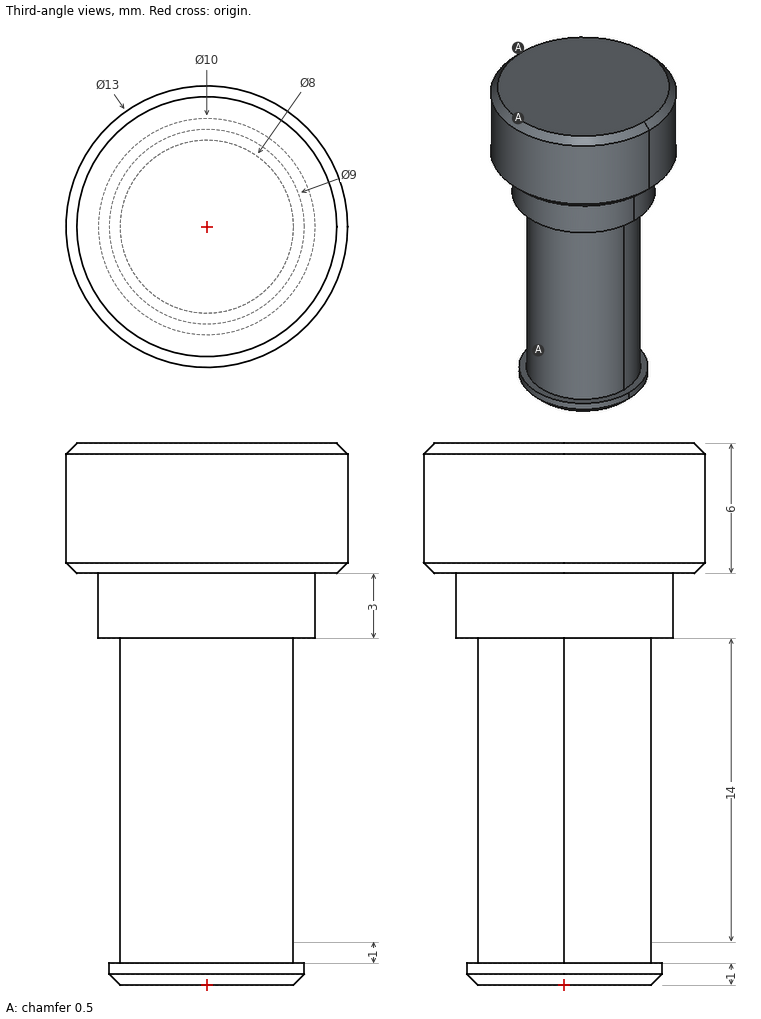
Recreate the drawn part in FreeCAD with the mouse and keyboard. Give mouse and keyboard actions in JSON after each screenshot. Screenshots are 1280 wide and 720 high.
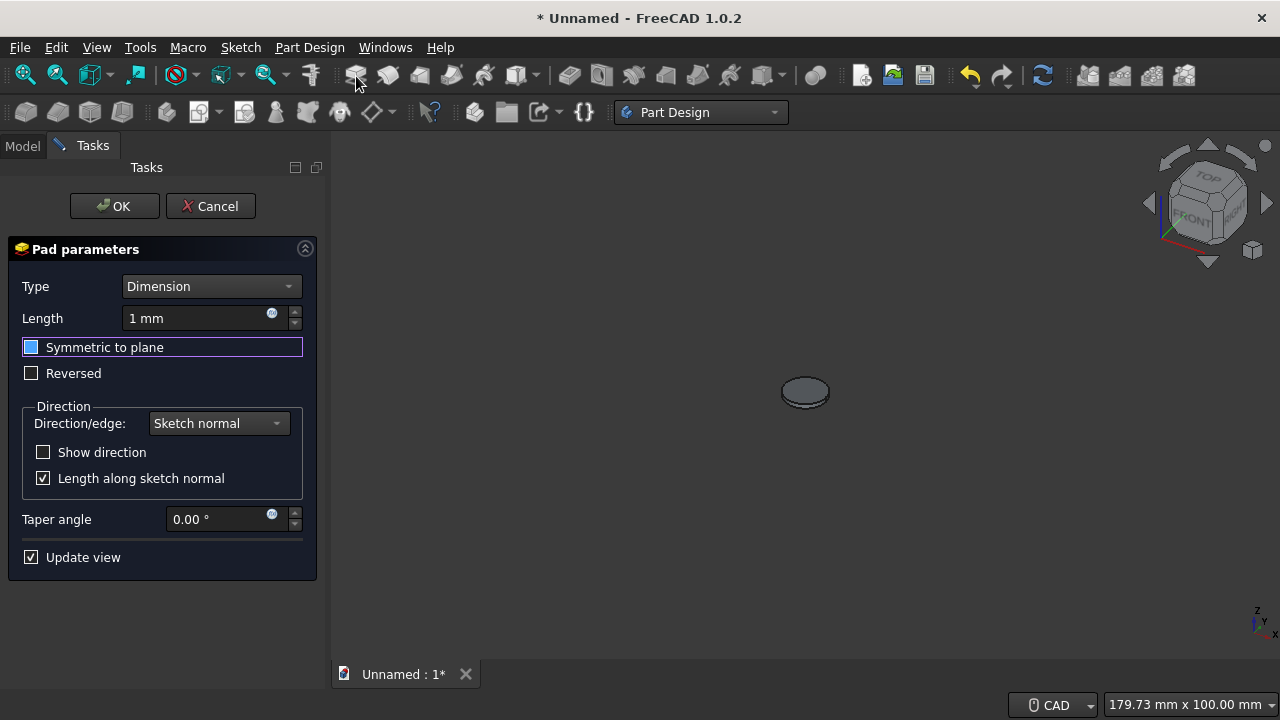
{"action": "left_click", "coordinate": [115, 206]}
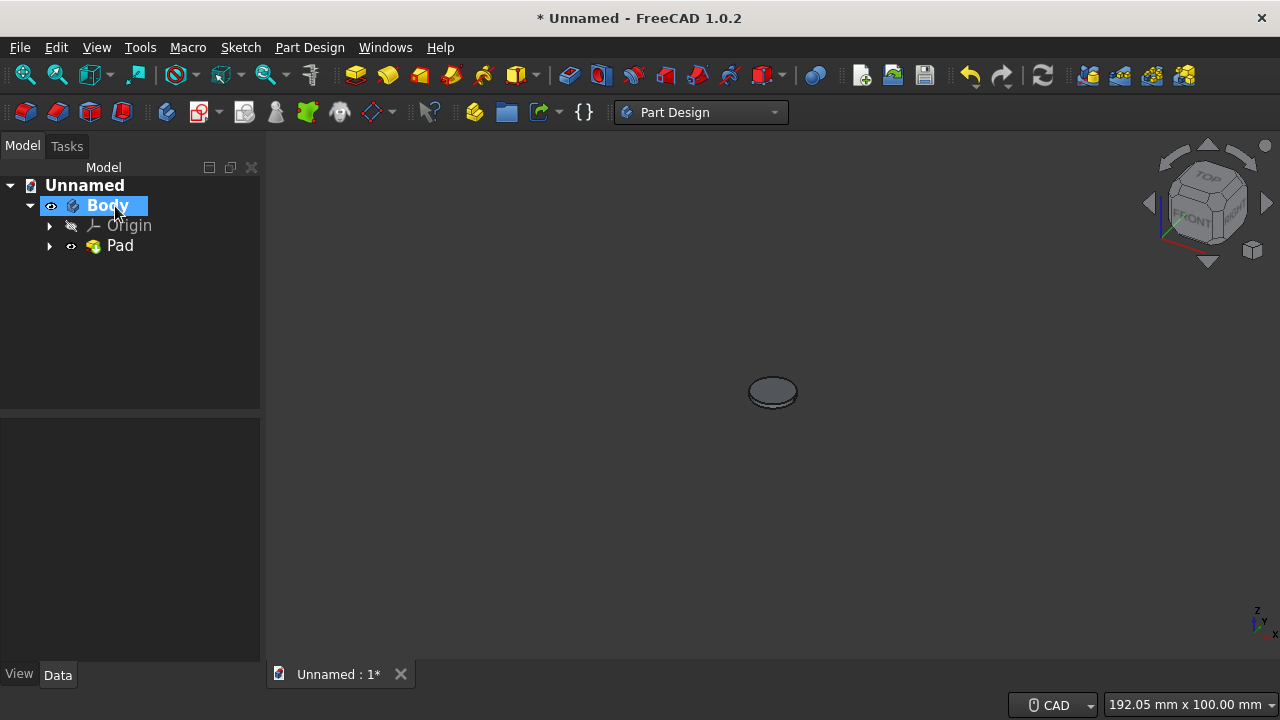
{"action": "left_click", "coordinate": [26, 76]}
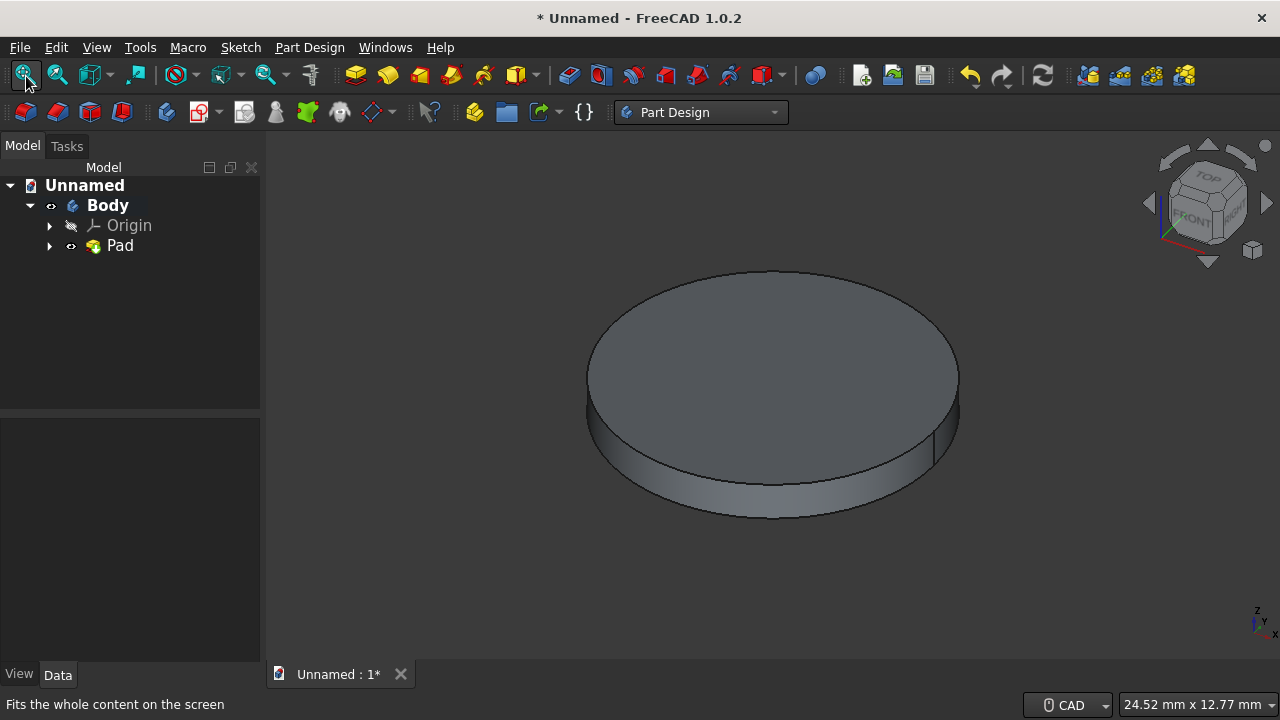
{"action": "left_click", "coordinate": [773, 377]}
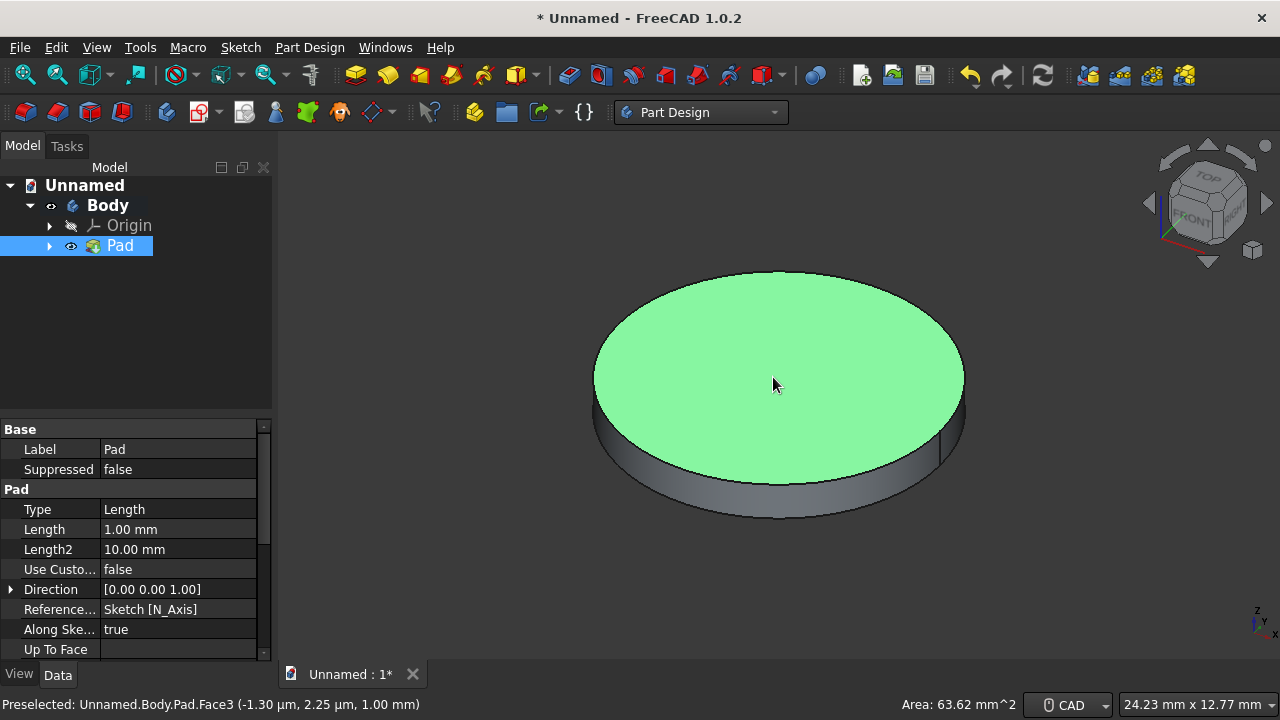
{"action": "left_click", "coordinate": [200, 112]}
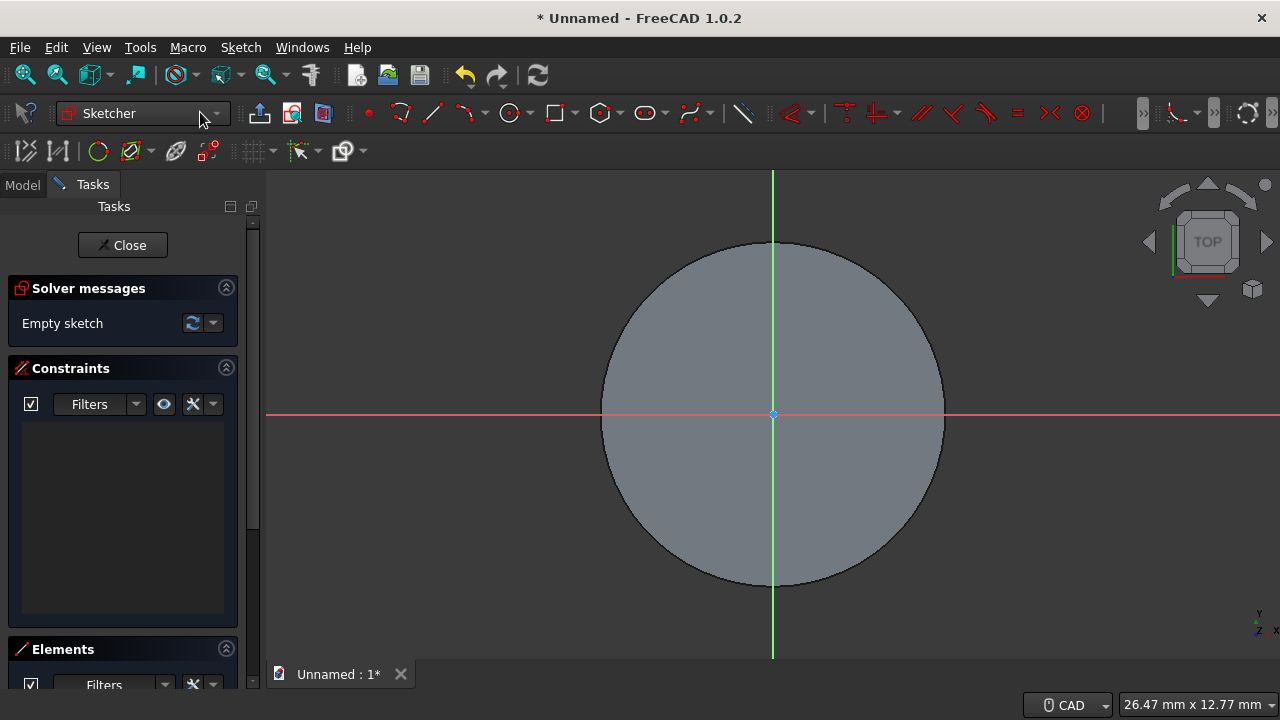
{"action": "left_click", "coordinate": [510, 114]}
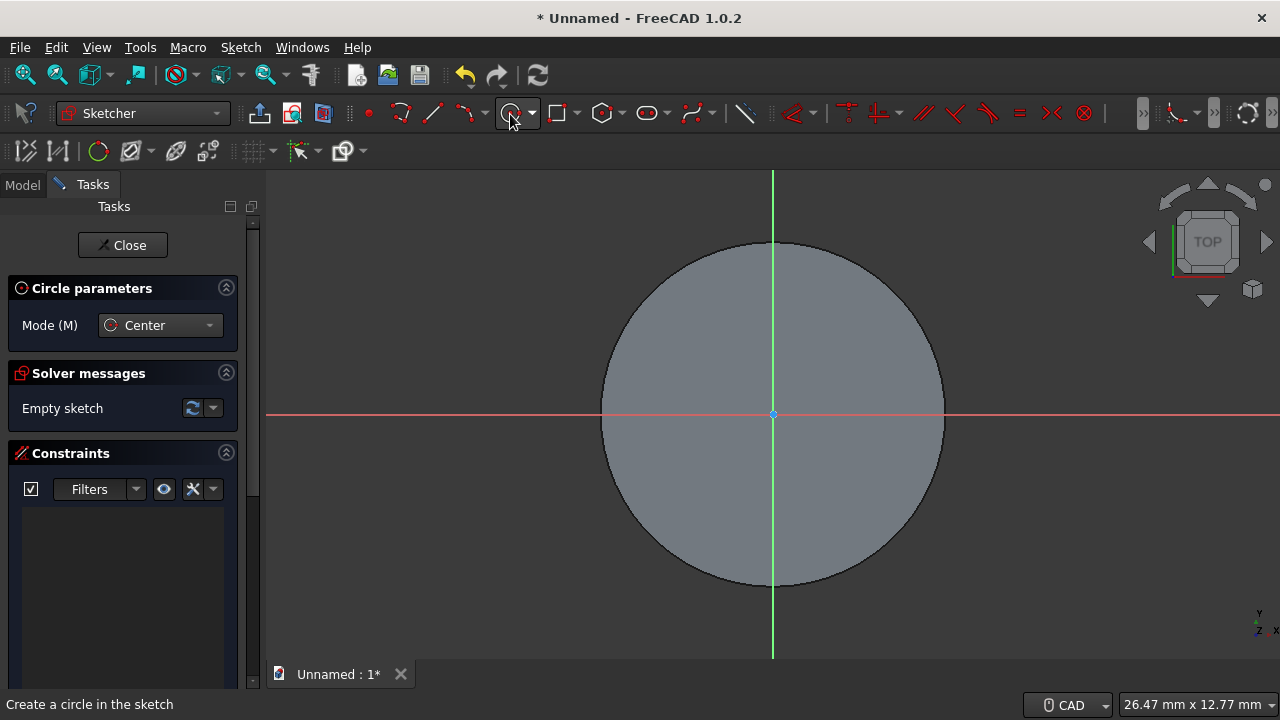
{"action": "left_click", "coordinate": [773, 414]}
{"action": "mouse_move", "coordinate": [881, 306]}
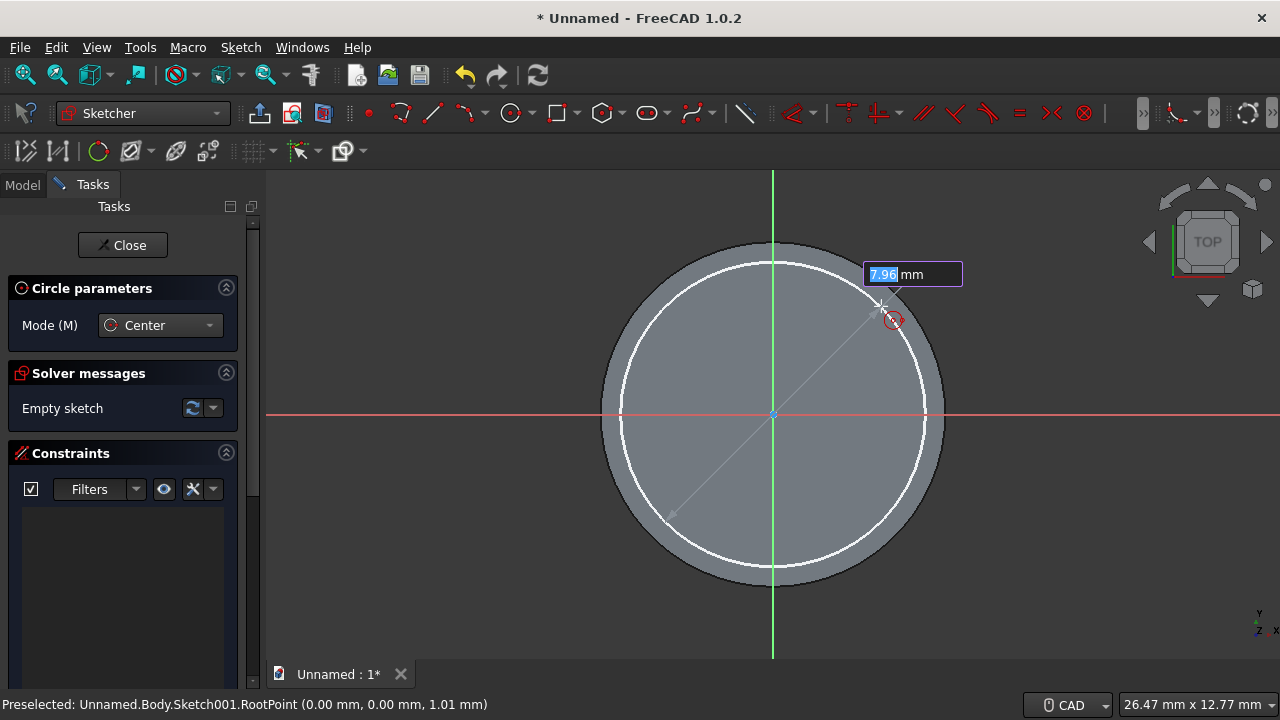
{"action": "type", "text": "8"}
{"action": "key", "text": "Return"}
{"action": "key", "text": "Escape"}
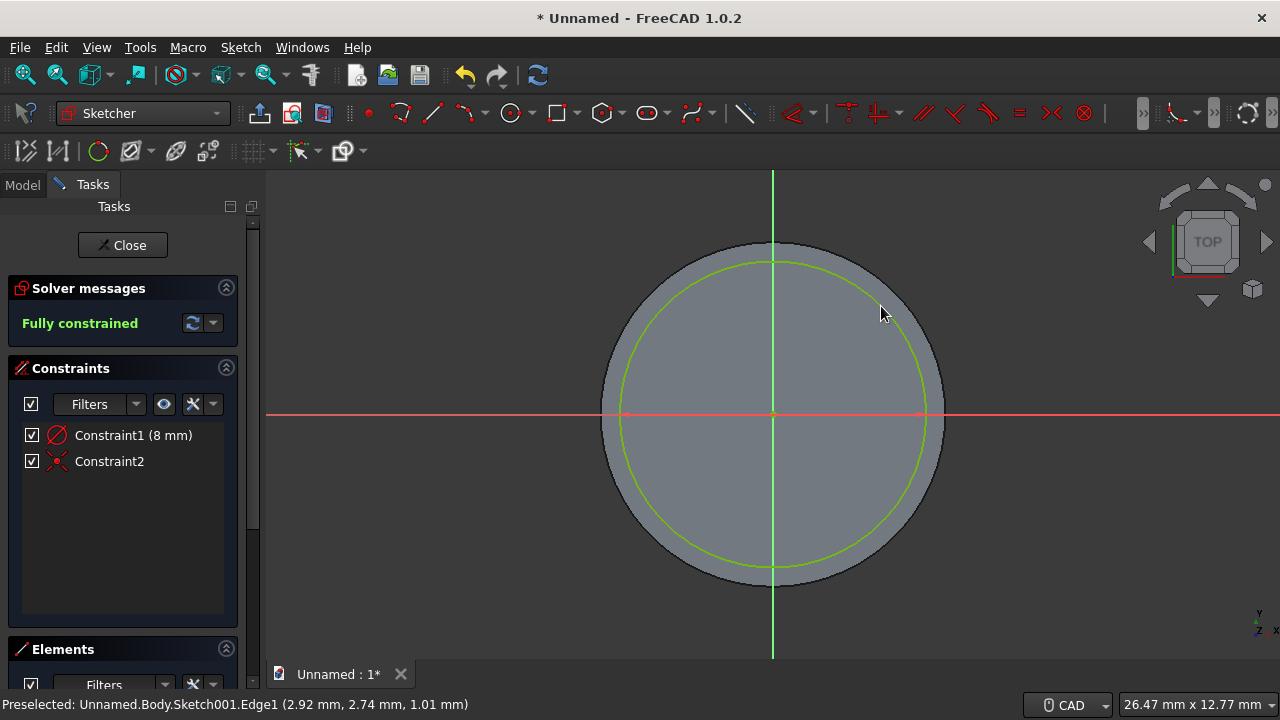
{"action": "left_click", "coordinate": [123, 245]}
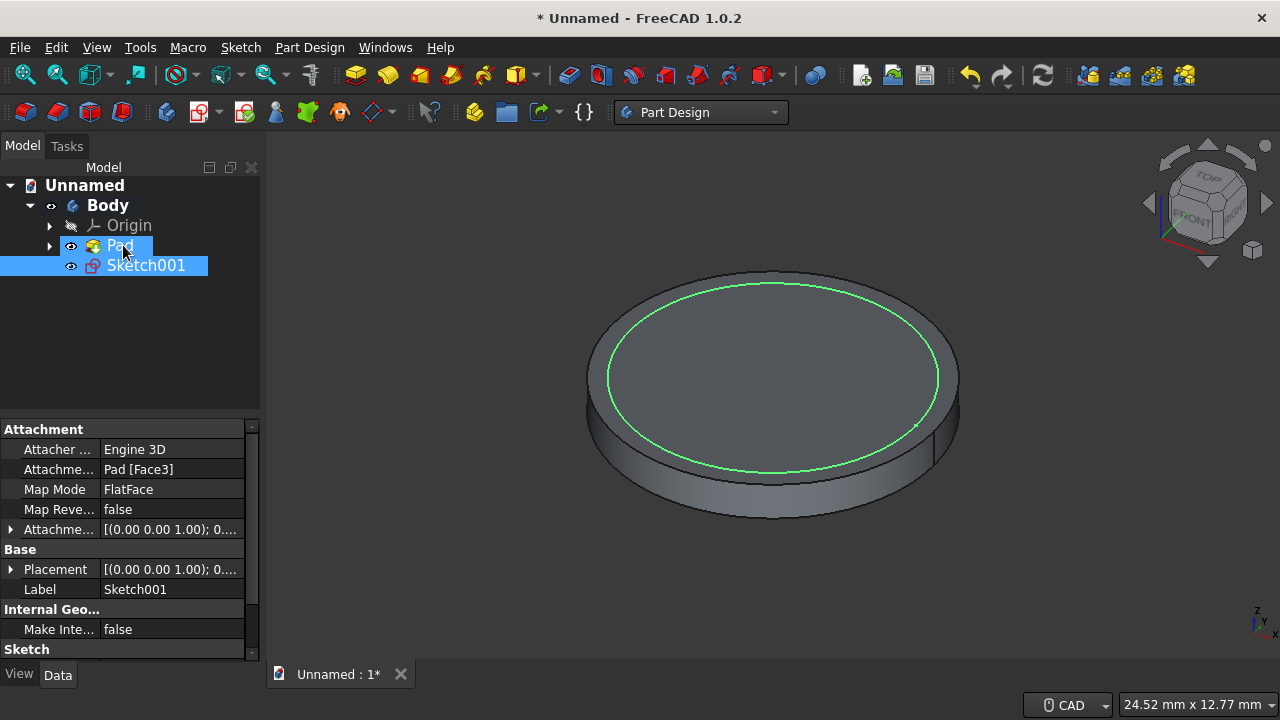
{"action": "left_click", "coordinate": [356, 76]}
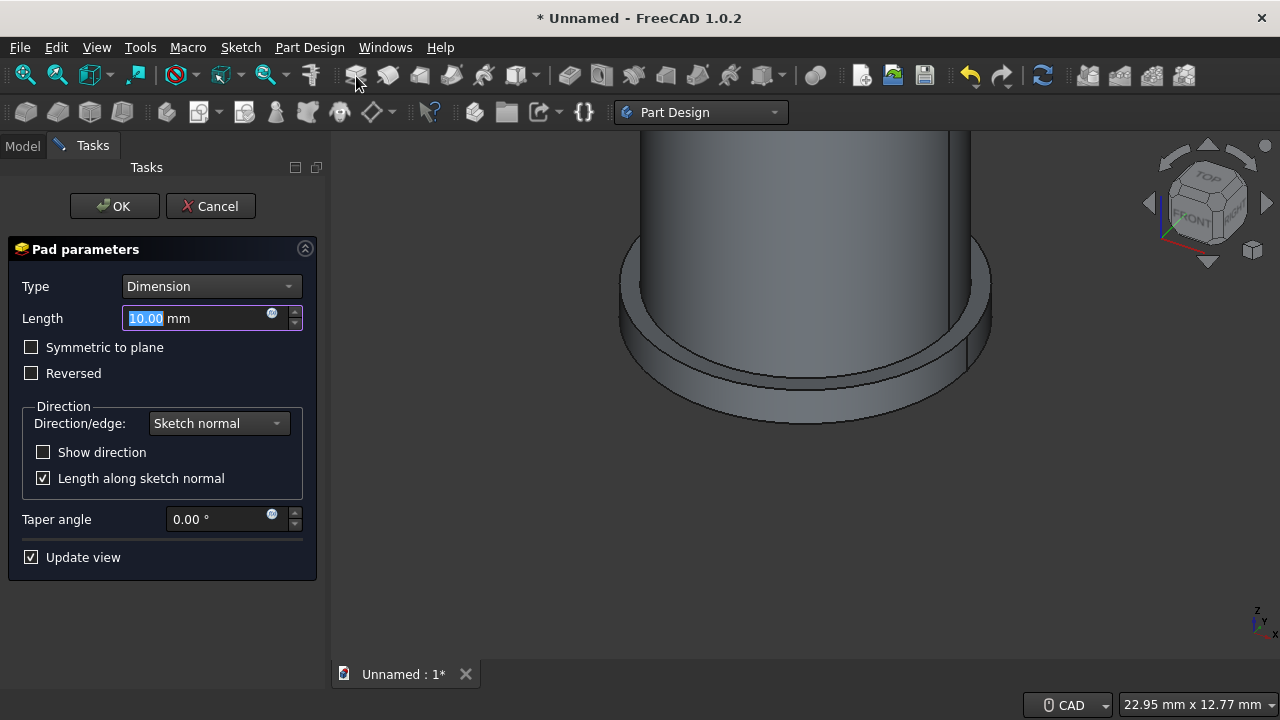
{"action": "type", "text": "1"}
{"action": "key", "text": "Tab"}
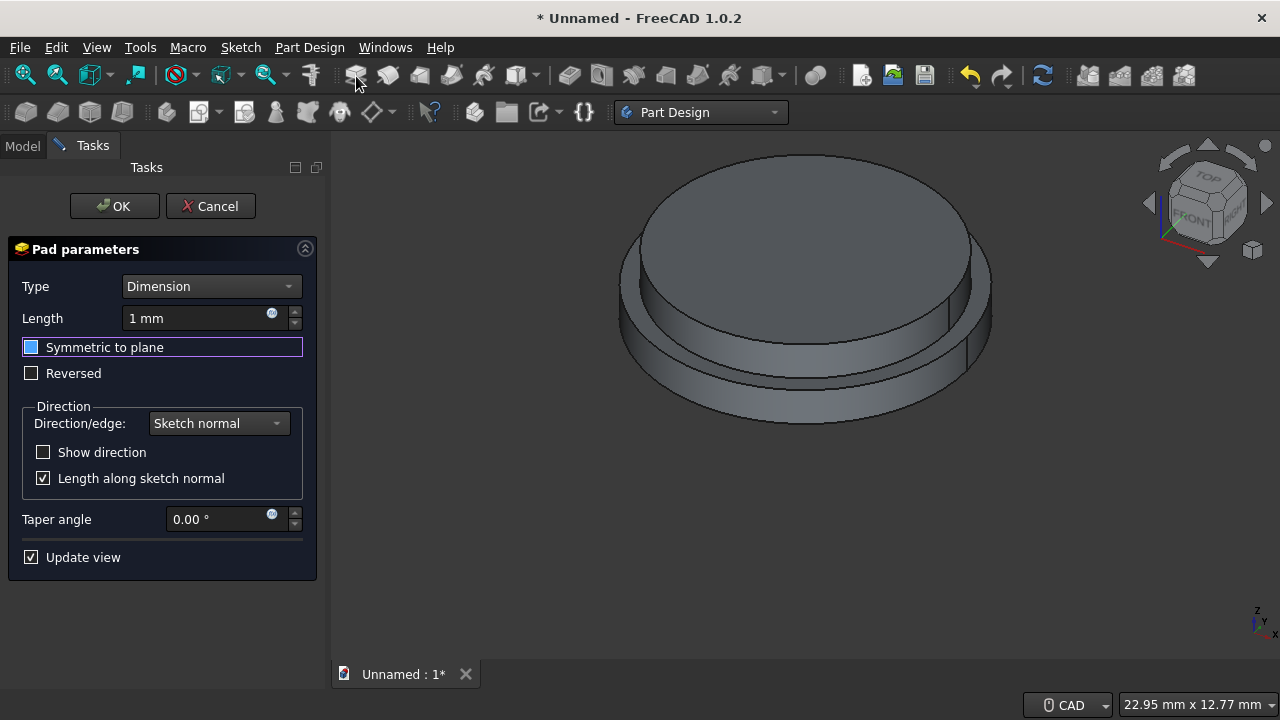
{"action": "left_click", "coordinate": [115, 206]}